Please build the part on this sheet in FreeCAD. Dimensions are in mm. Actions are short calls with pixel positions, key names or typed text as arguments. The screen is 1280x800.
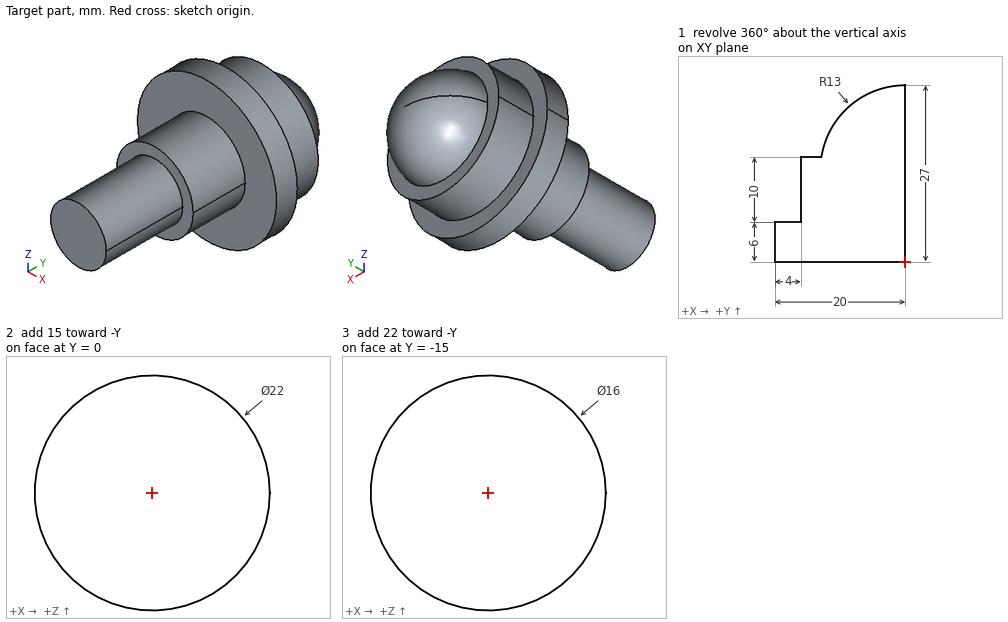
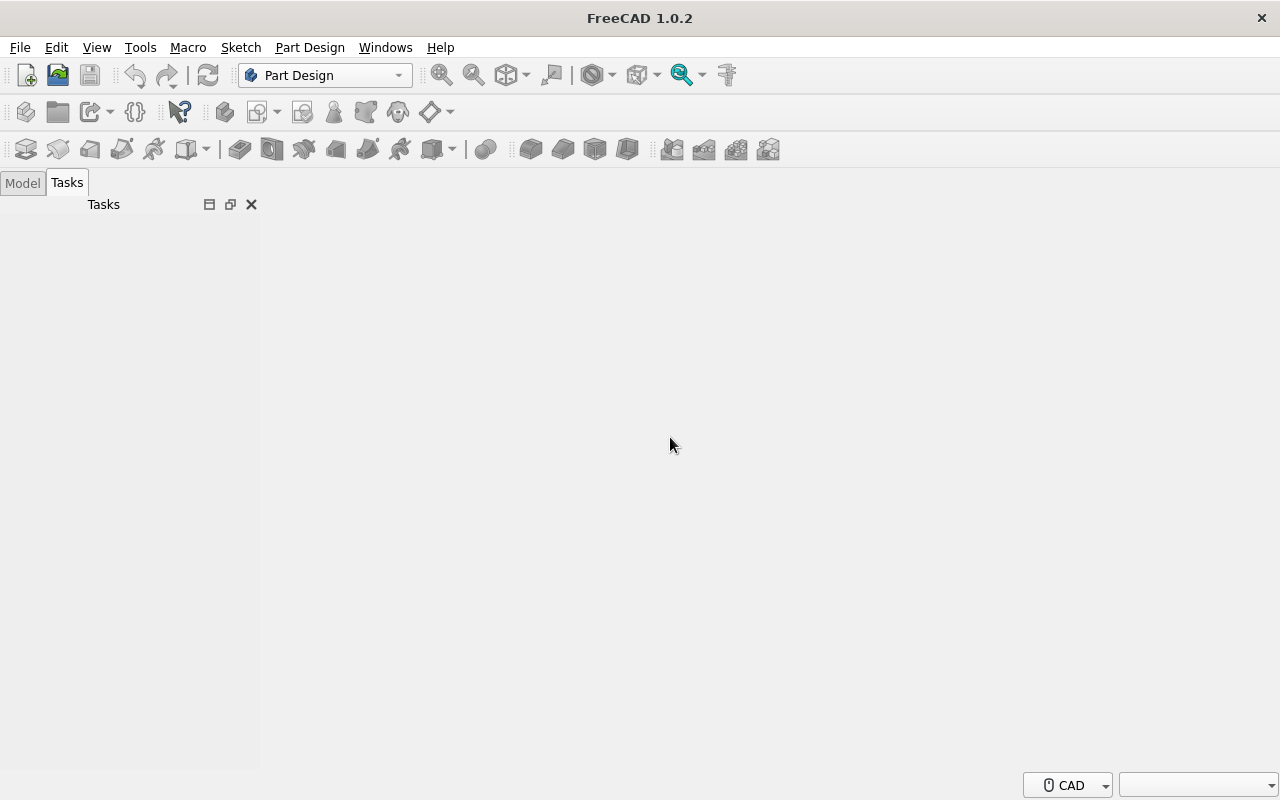
click(26, 76)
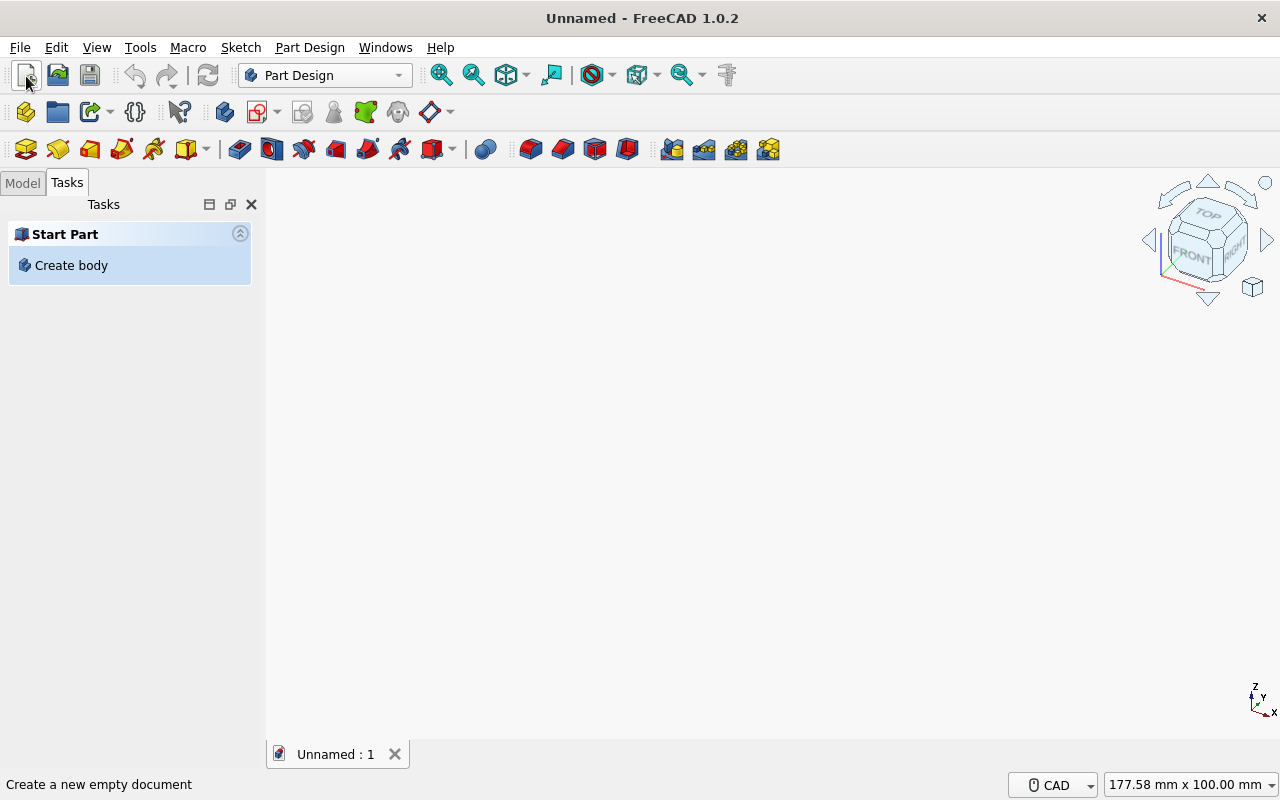
click(258, 112)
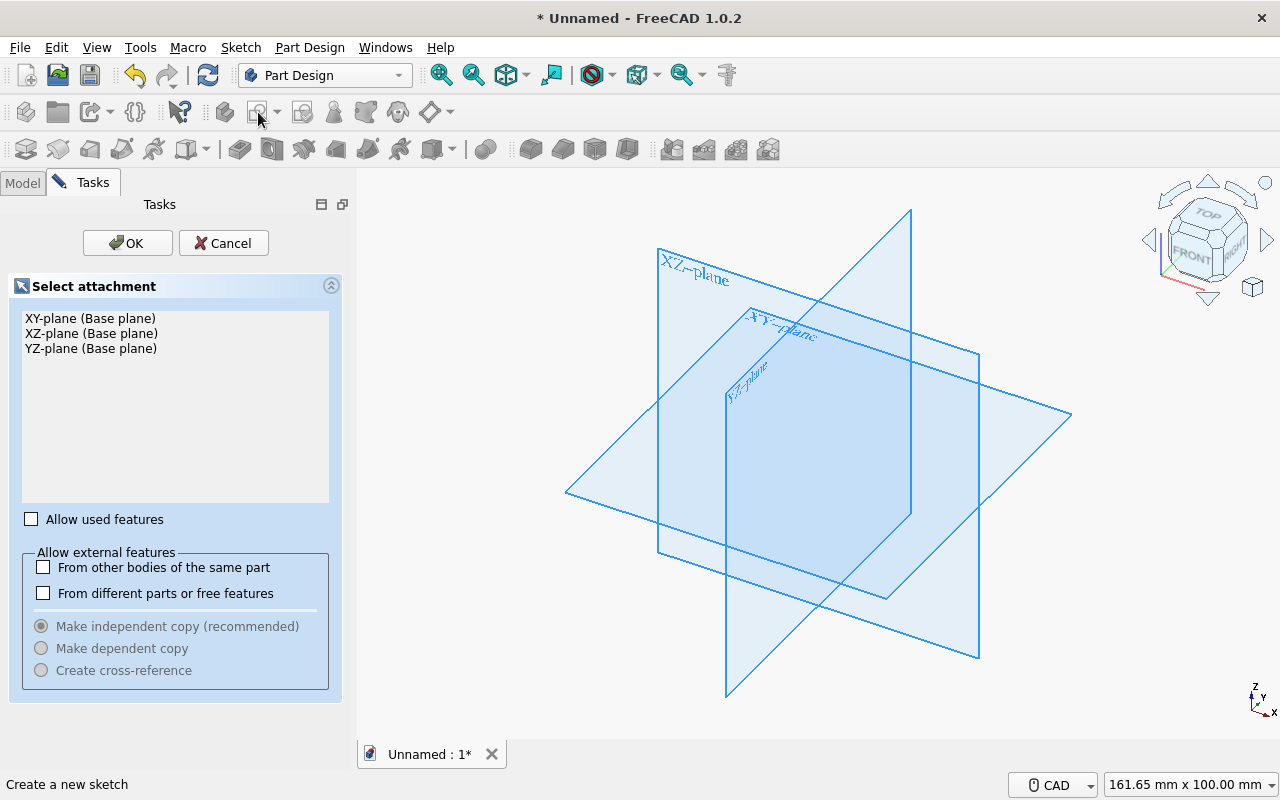
click(82, 318)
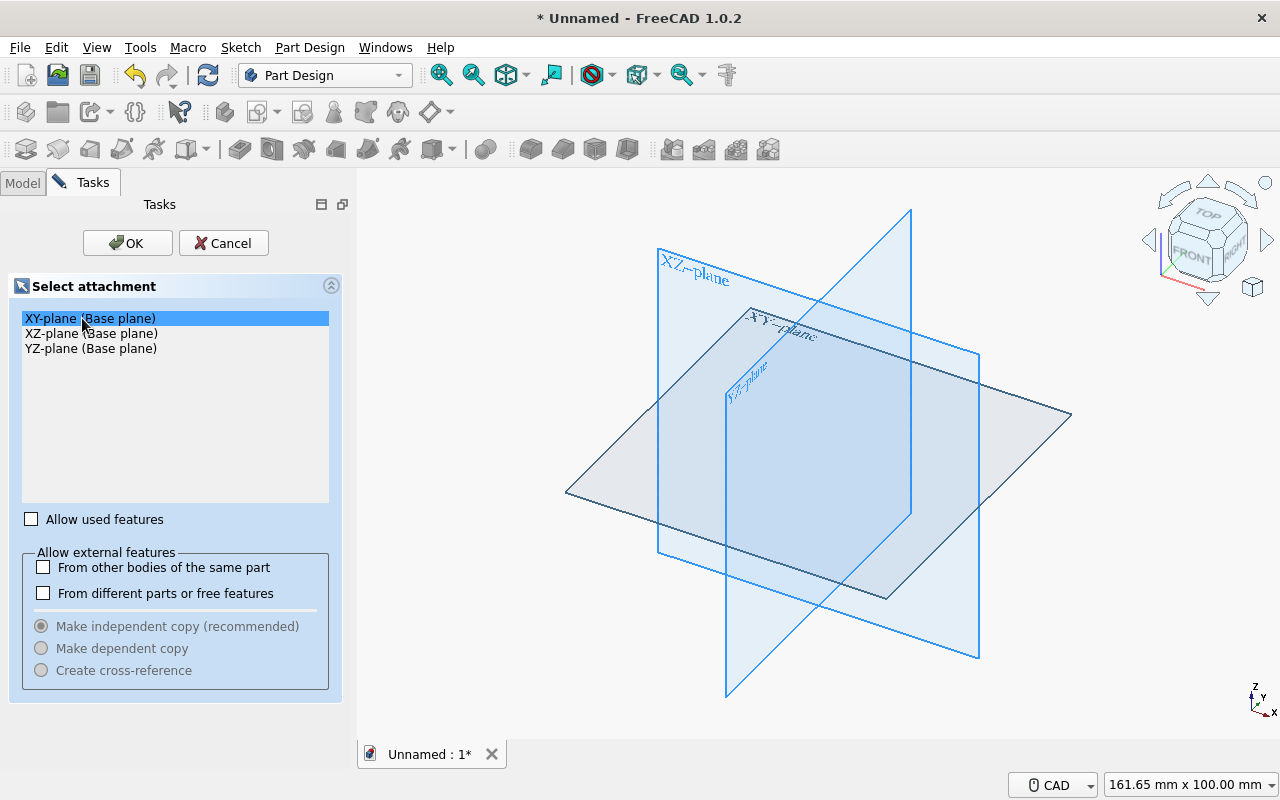
click(128, 243)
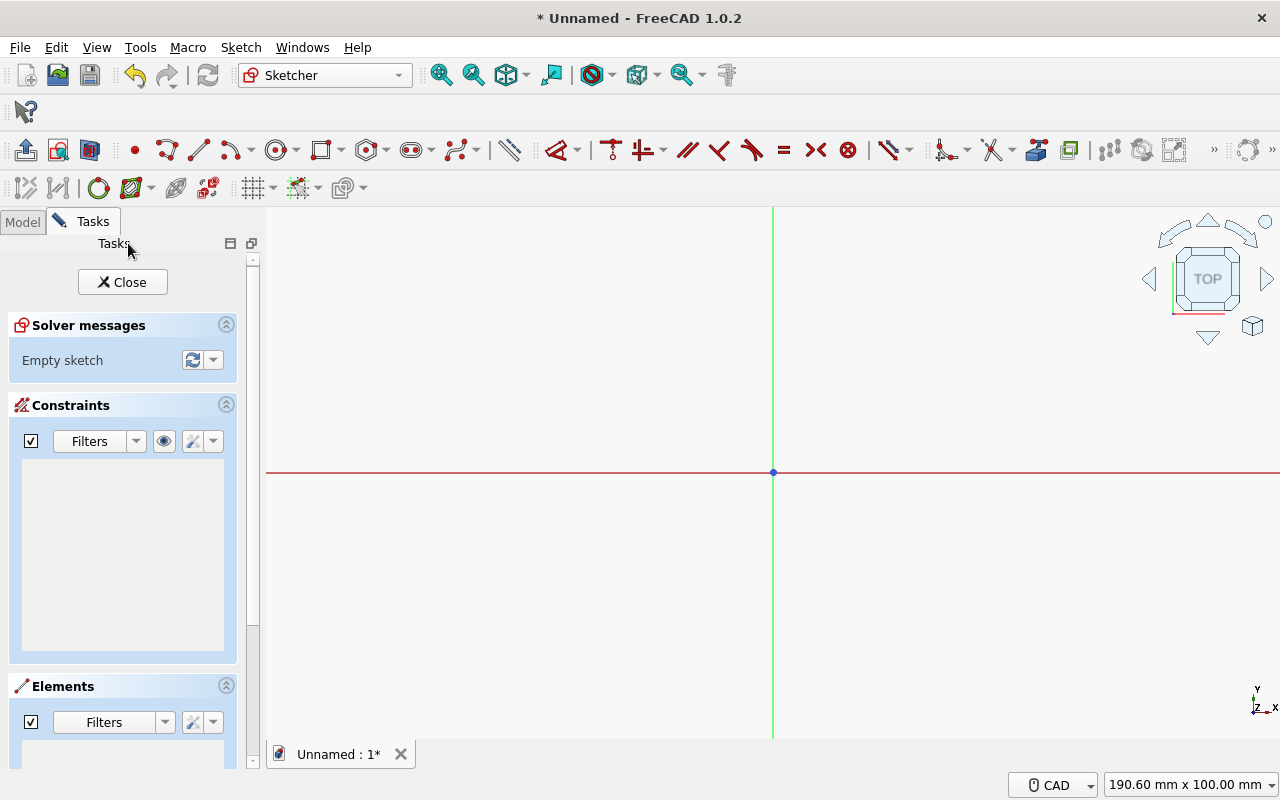
scroll(732, 343, up, 4)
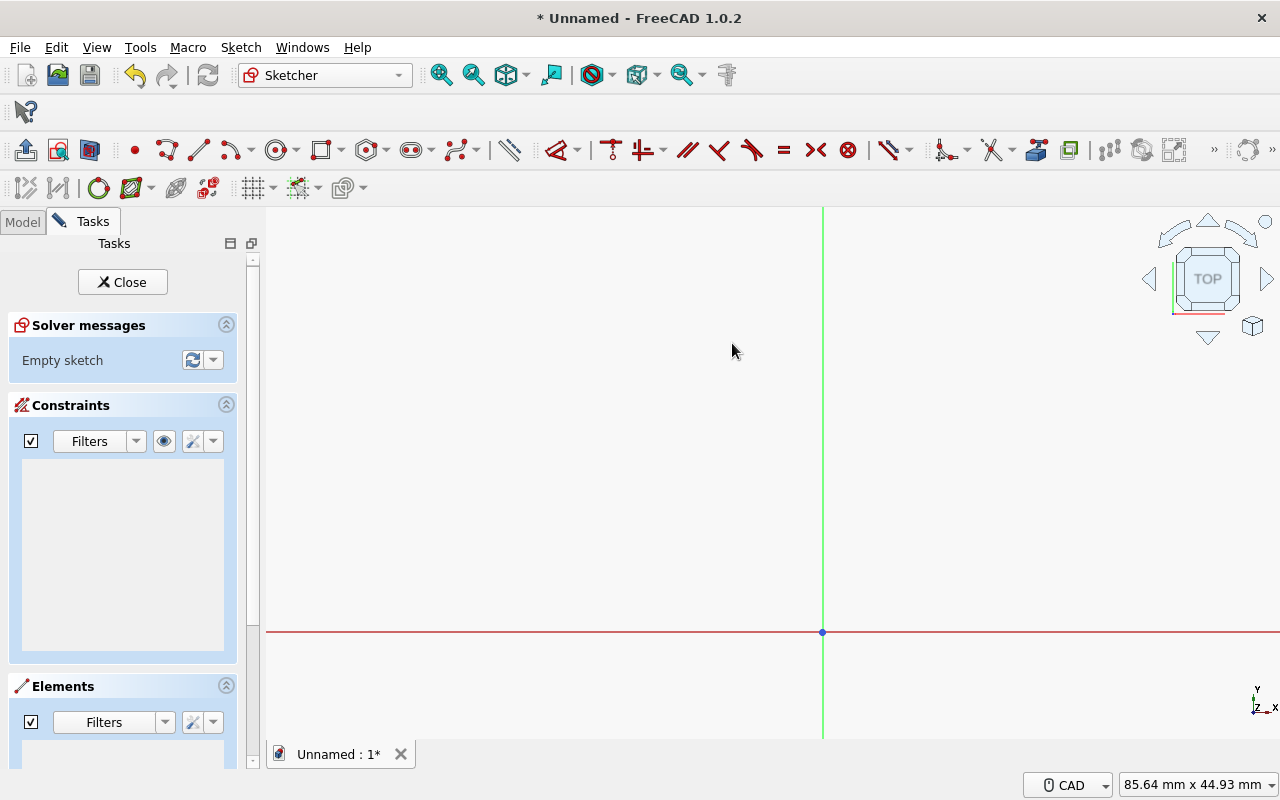
click(168, 150)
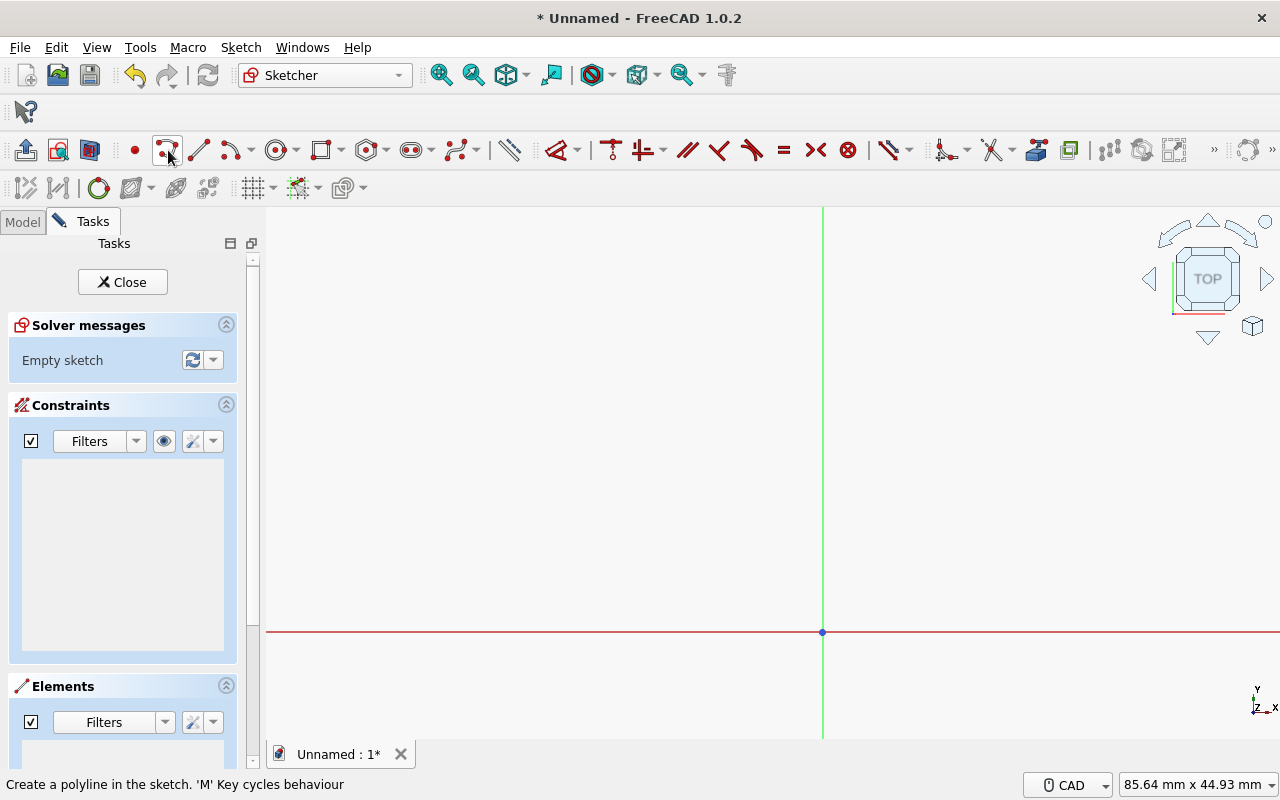
click(671, 443)
click(633, 443)
click(633, 561)
click(586, 561)
click(586, 632)
click(823, 632)
click(814, 312)
right_click(814, 312)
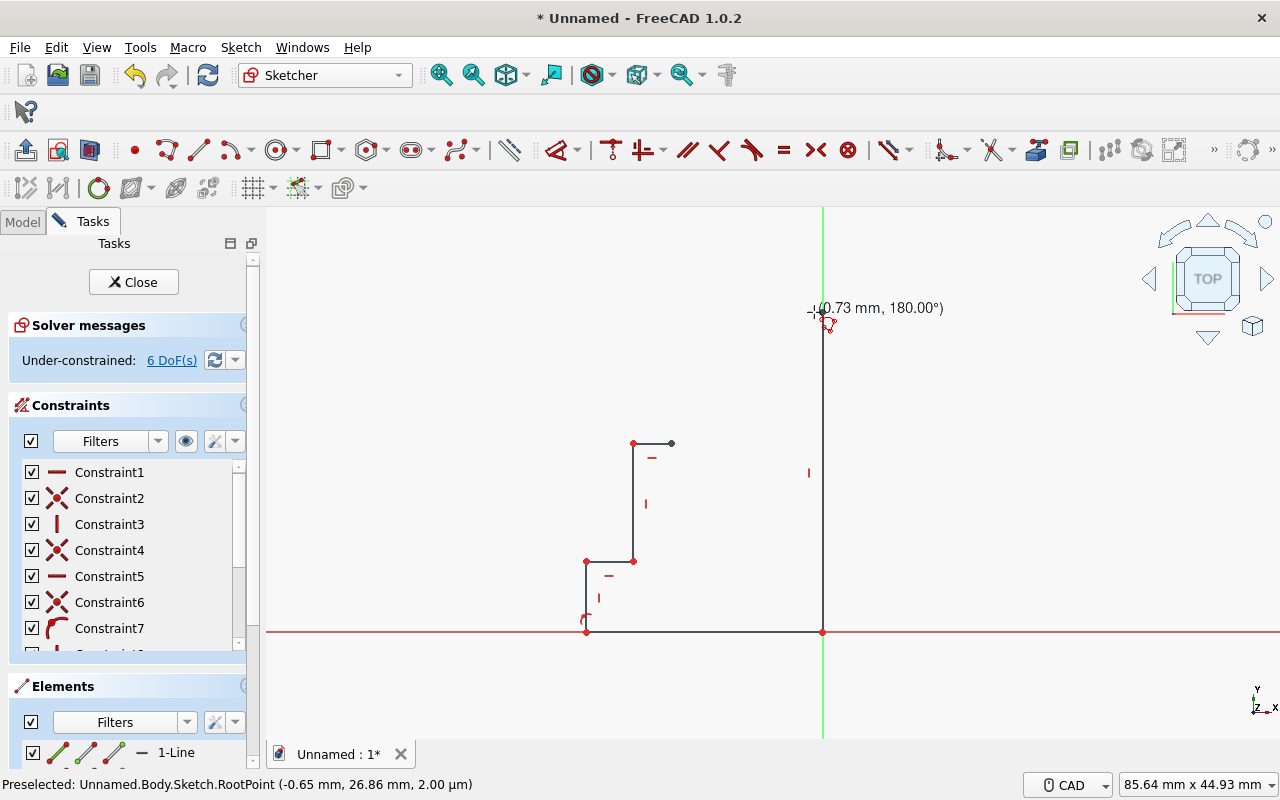
key(g)
key(3)
key(a)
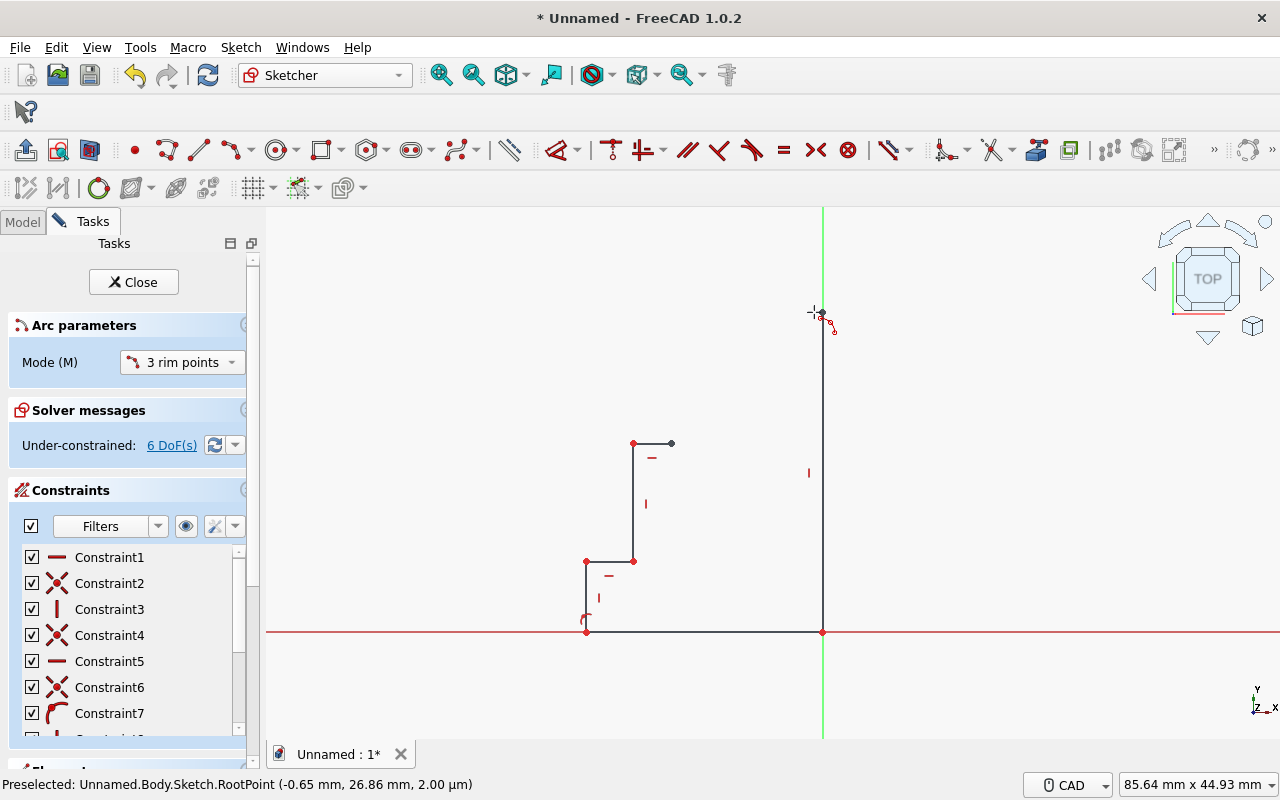
click(823, 313)
click(671, 444)
click(723, 349)
key(Escape)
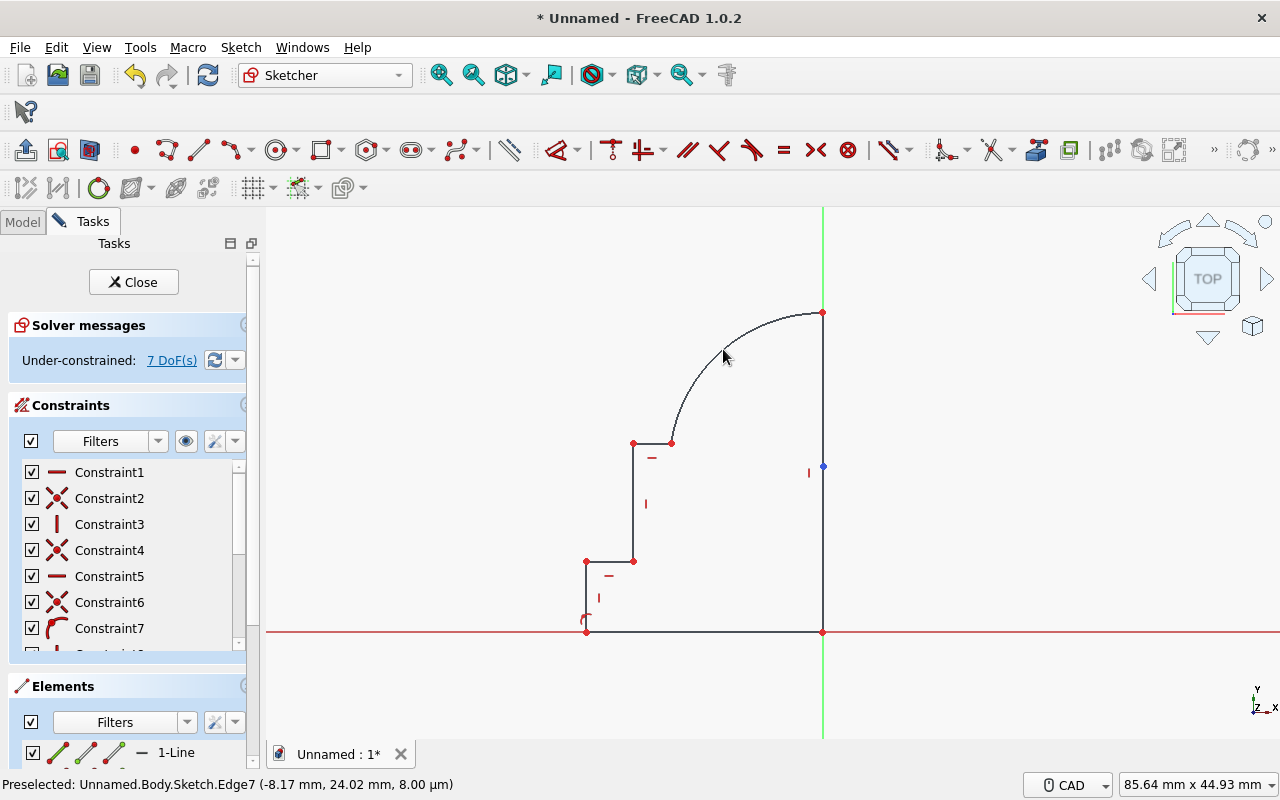
click(823, 467)